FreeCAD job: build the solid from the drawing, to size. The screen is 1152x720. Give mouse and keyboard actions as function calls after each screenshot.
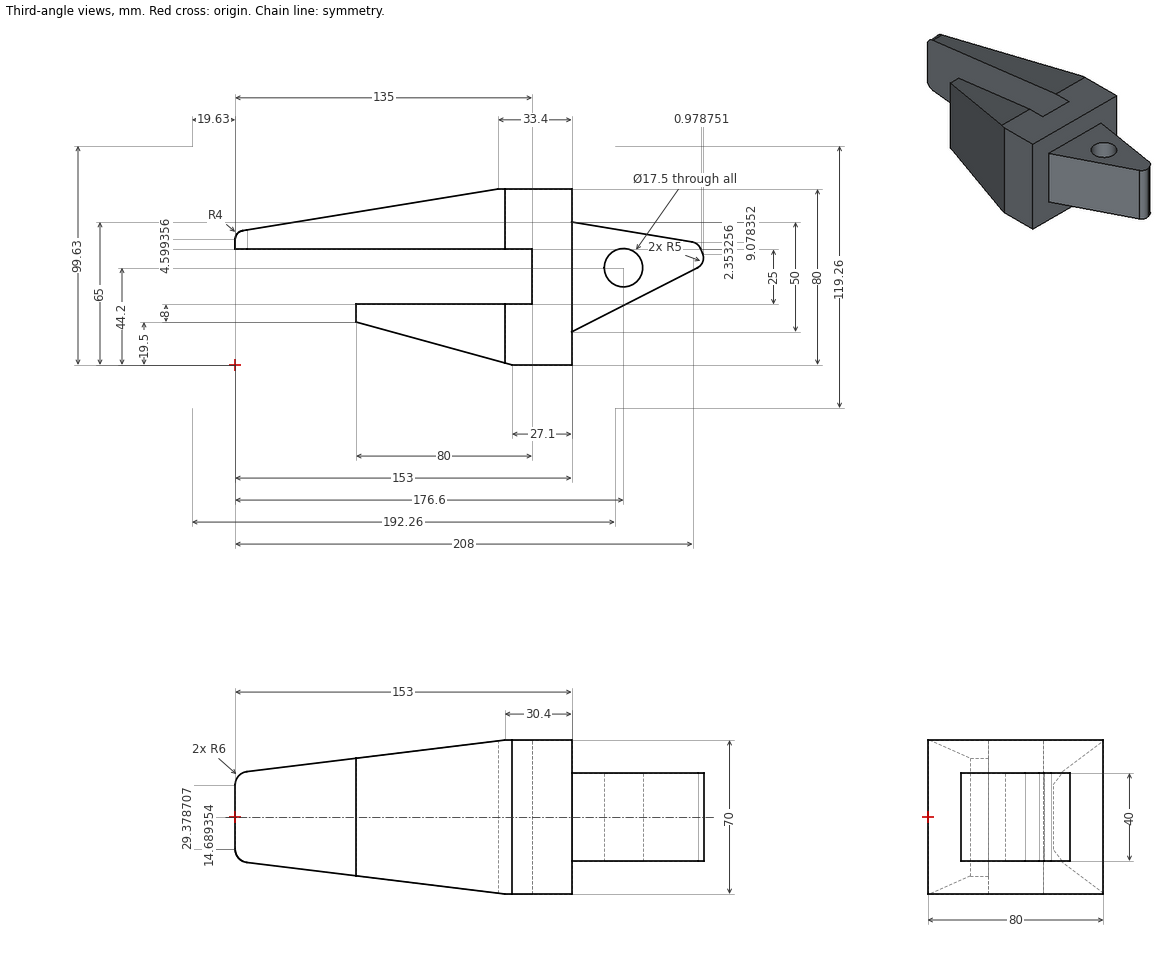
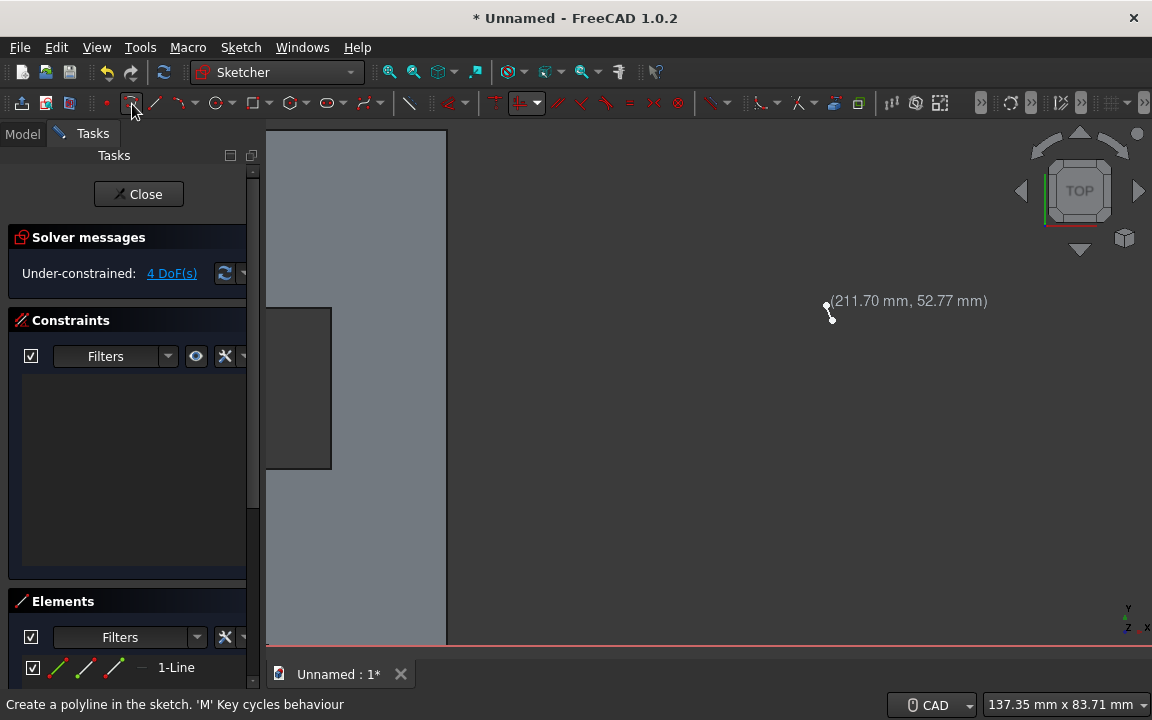
click(801, 286)
click(447, 227)
click(447, 550)
click(817, 361)
right_click(817, 361)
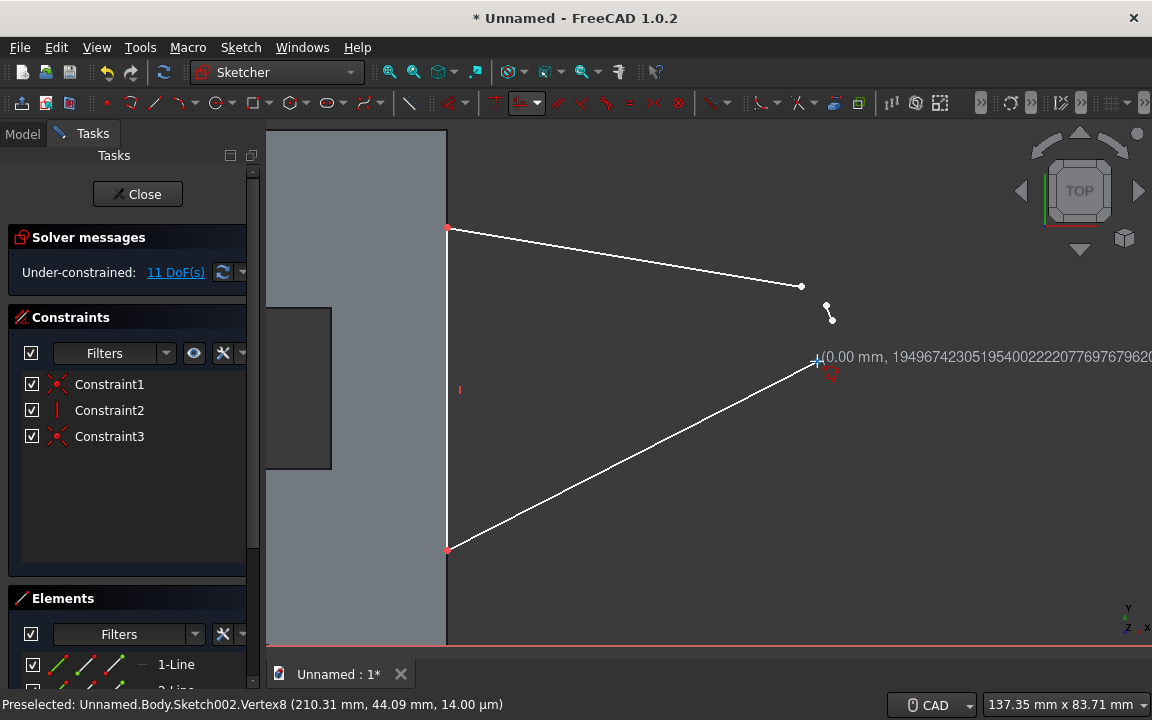
click(180, 104)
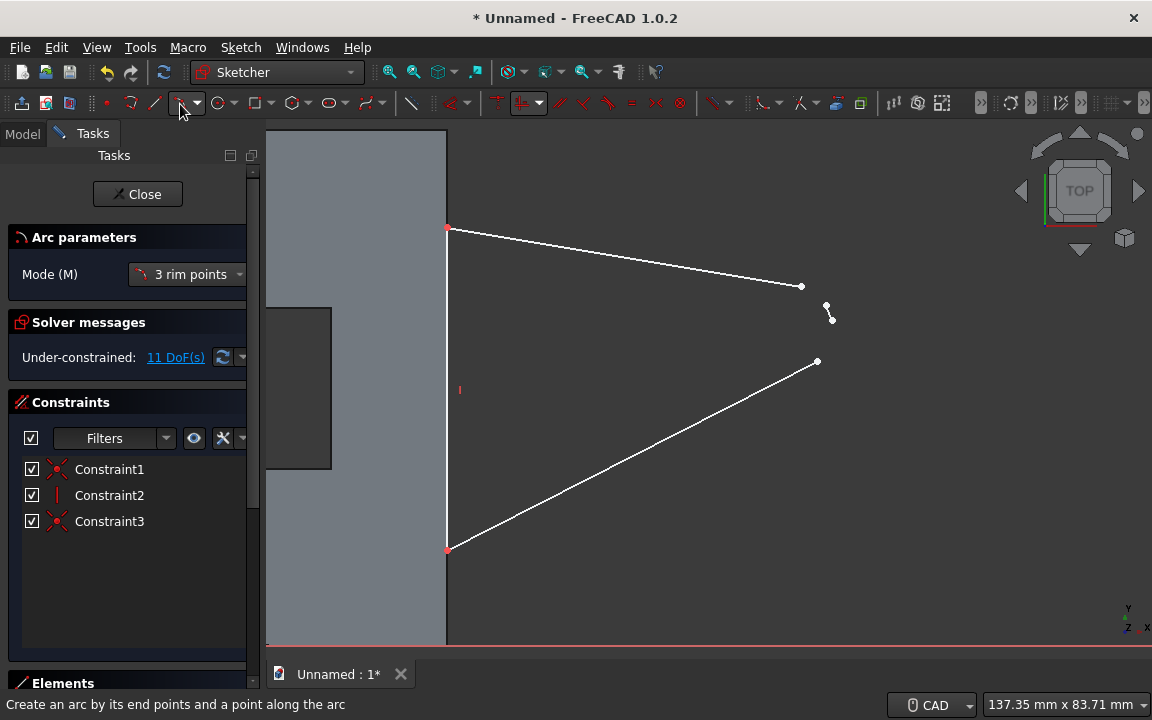
scroll(826, 305, up, 4)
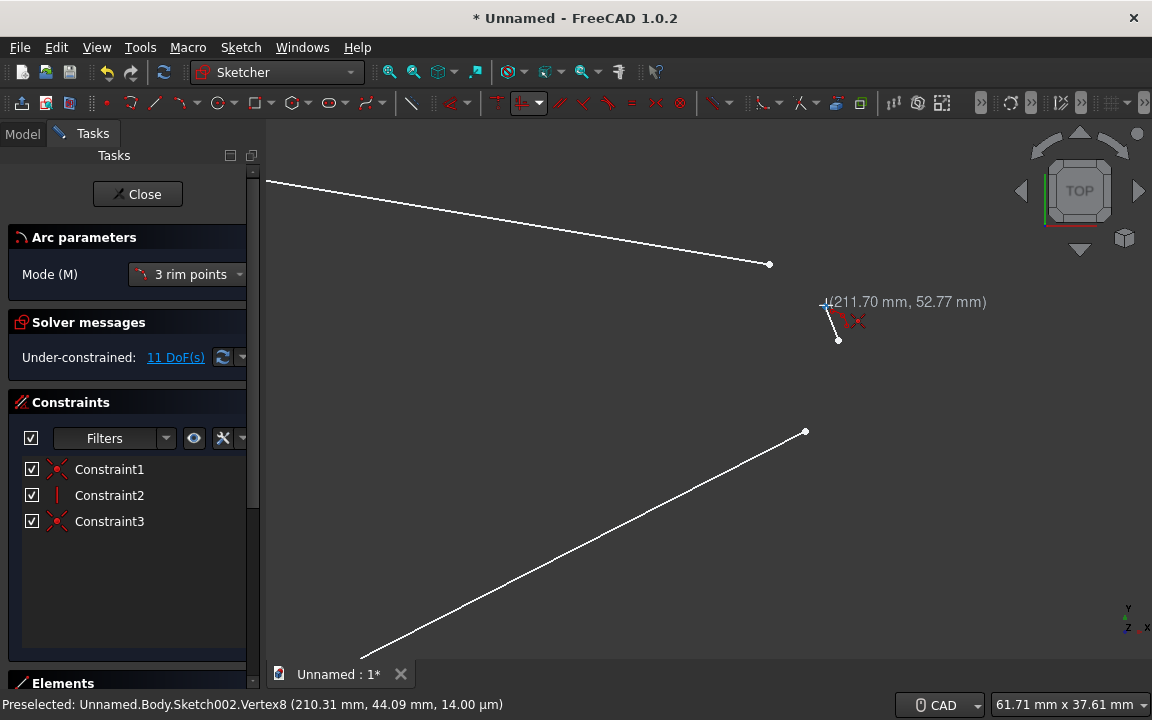
click(825, 307)
click(770, 265)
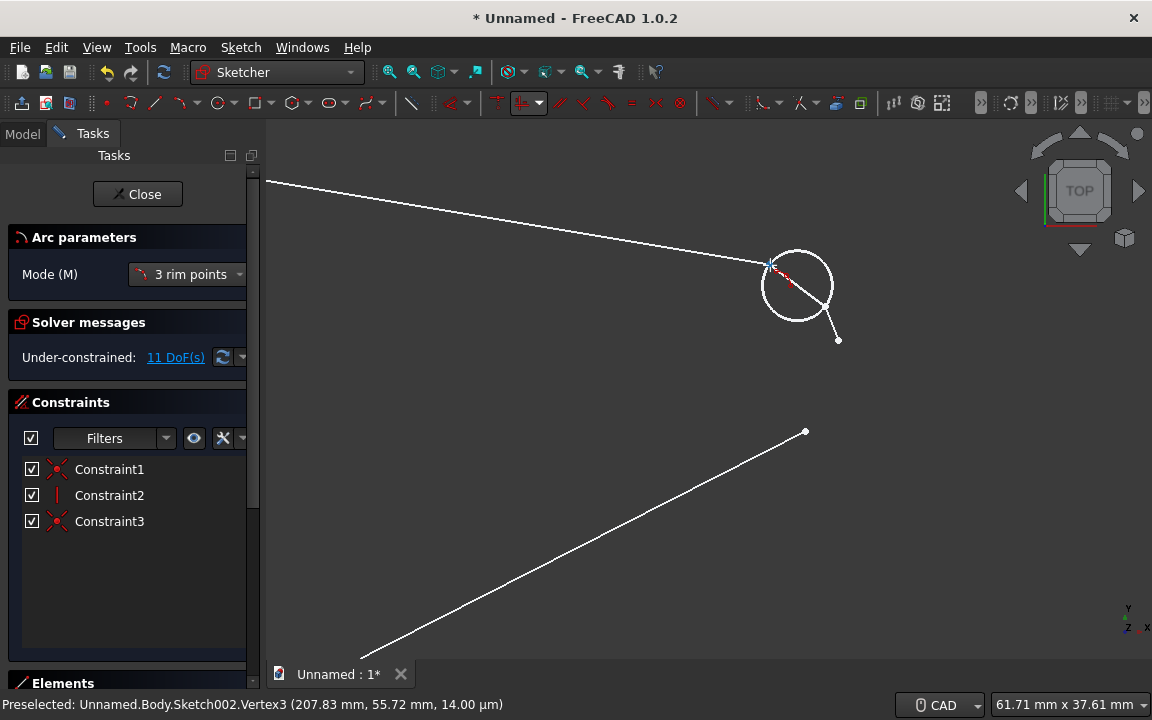
scroll(803, 276, up, 3)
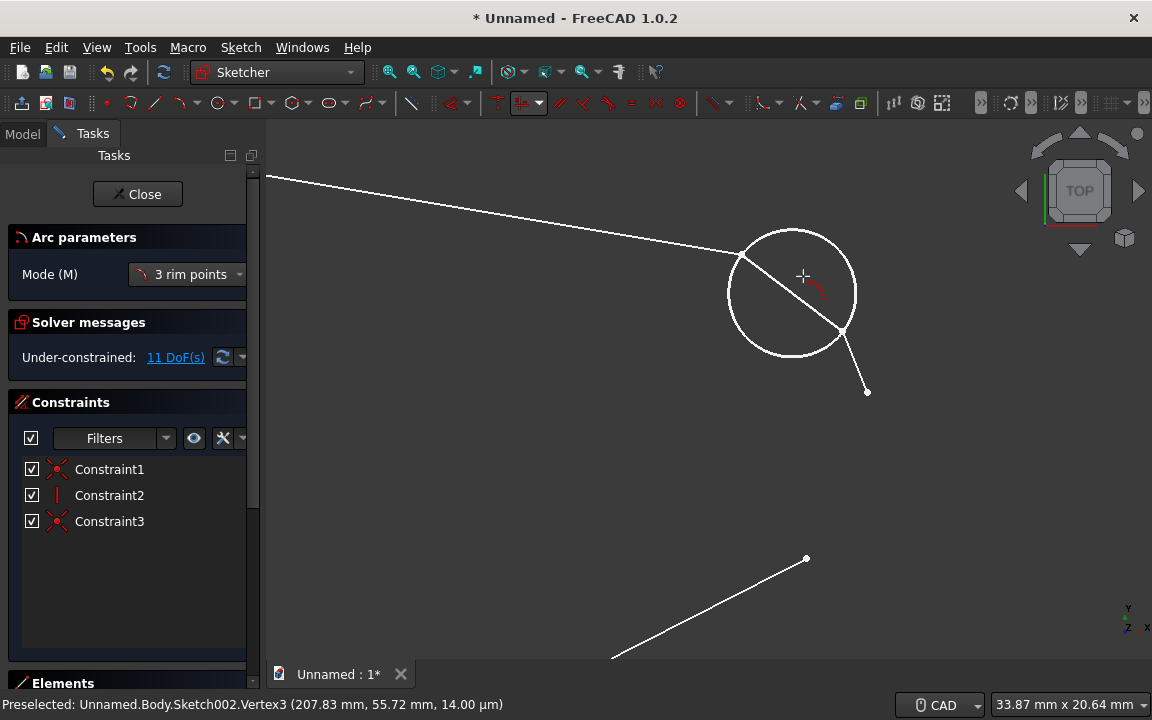
click(802, 276)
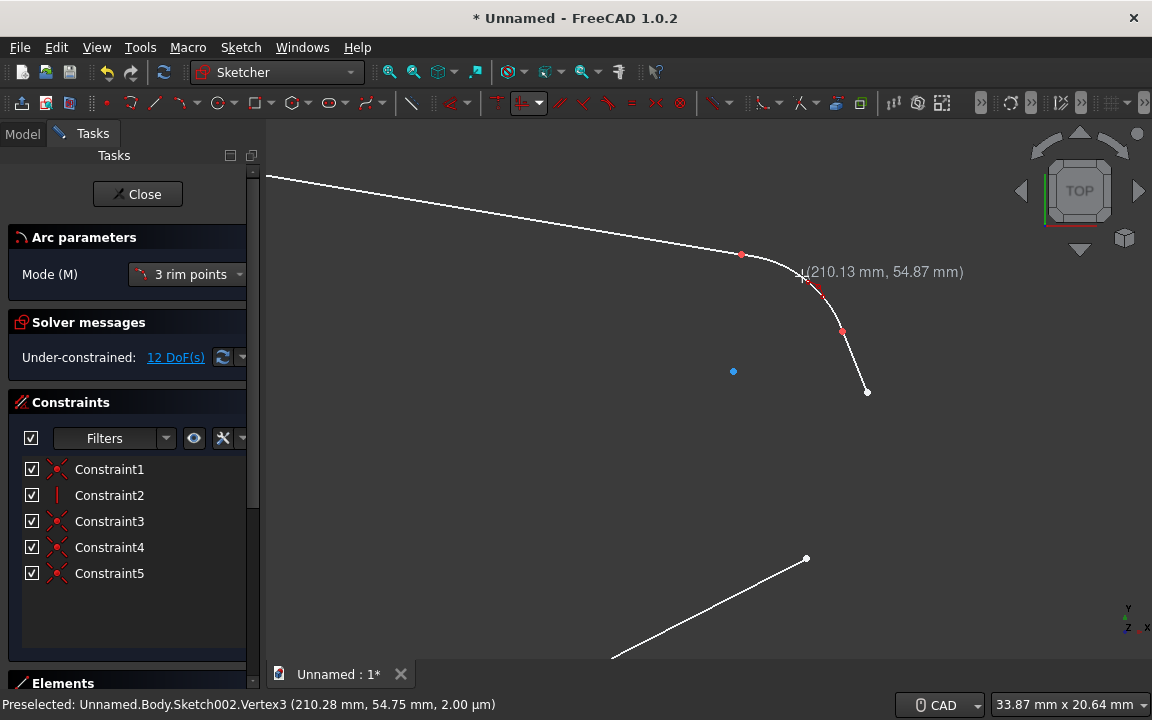
scroll(821, 298, down, 7)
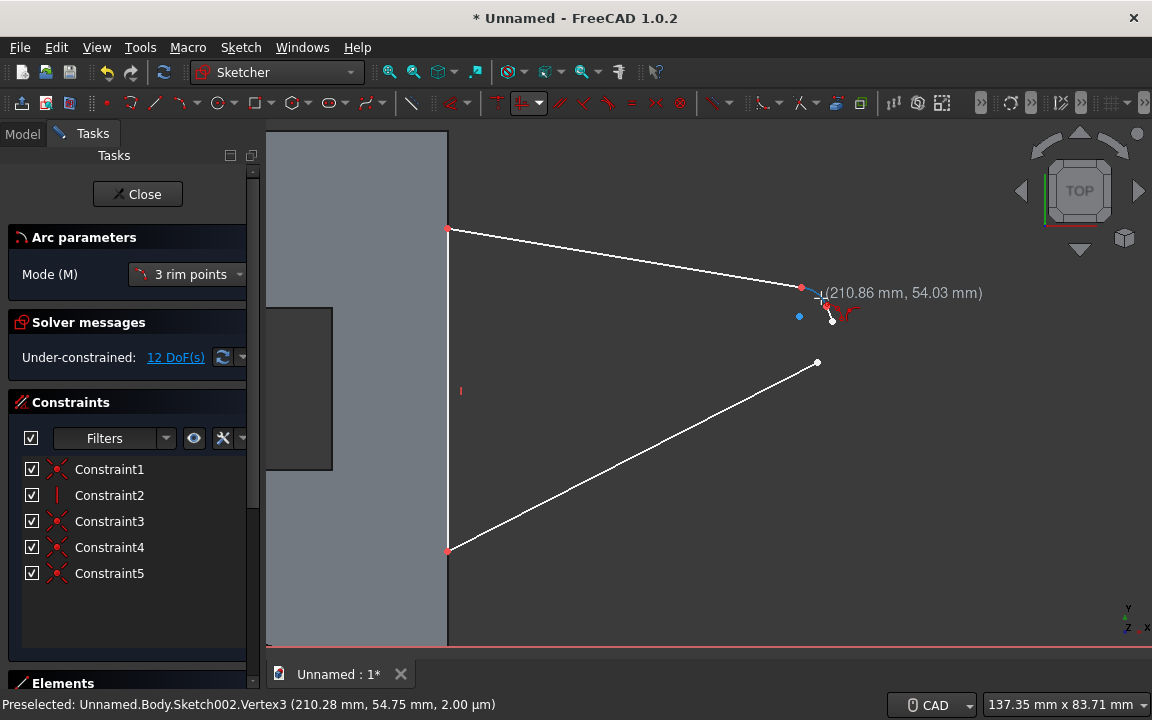
click(818, 363)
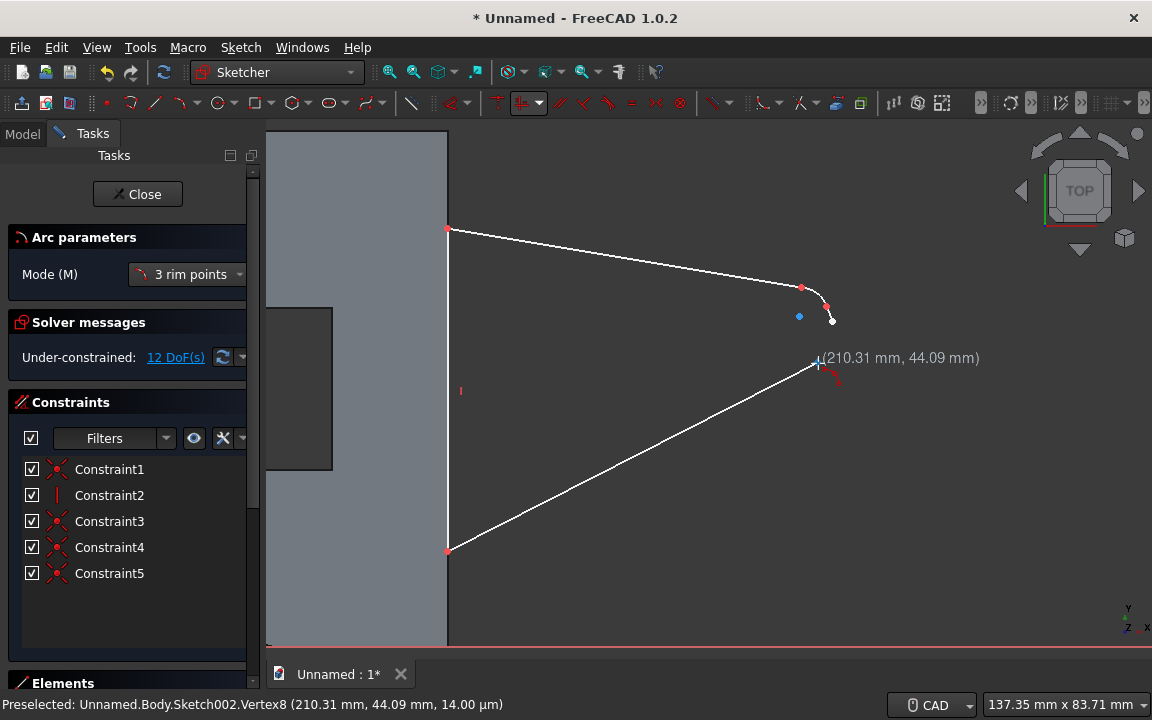
scroll(833, 321, up, 4)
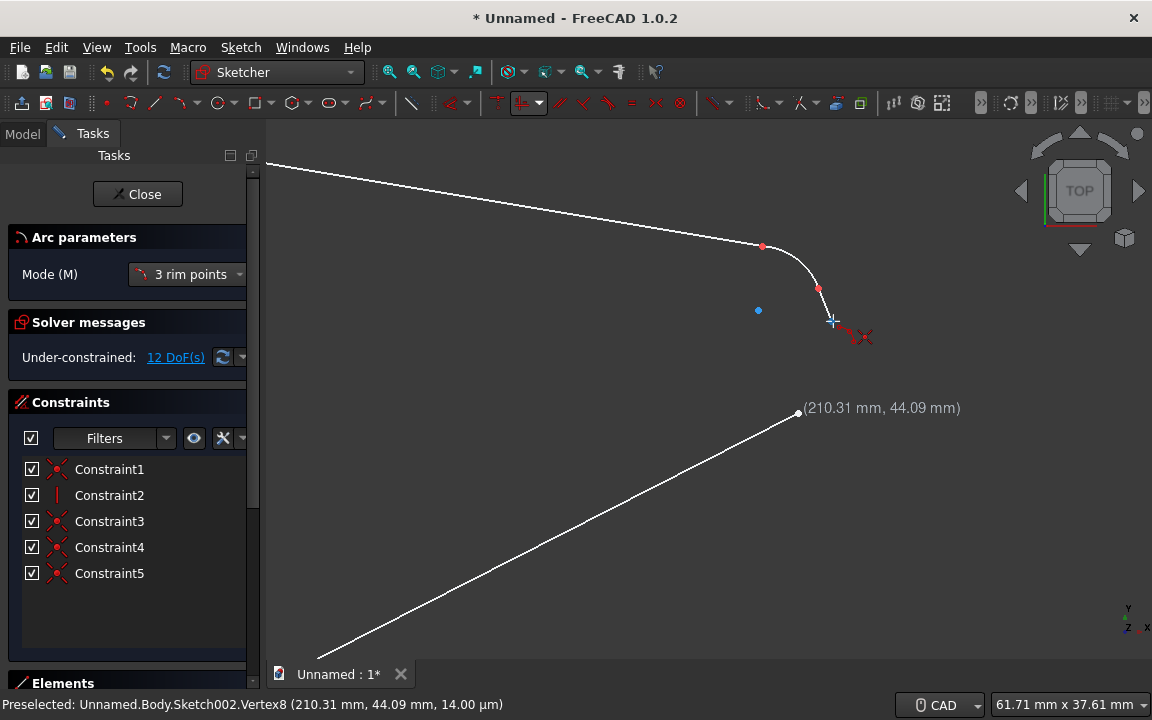
click(832, 322)
click(833, 373)
key(Escape)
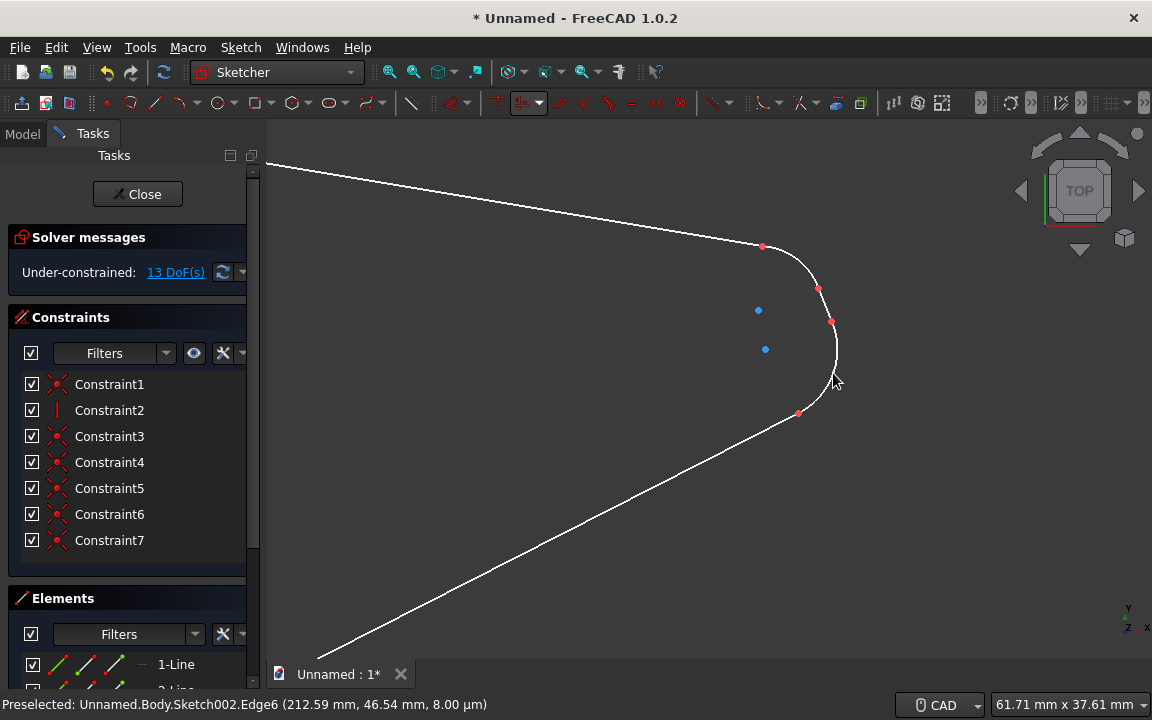
scroll(828, 312, up, 2)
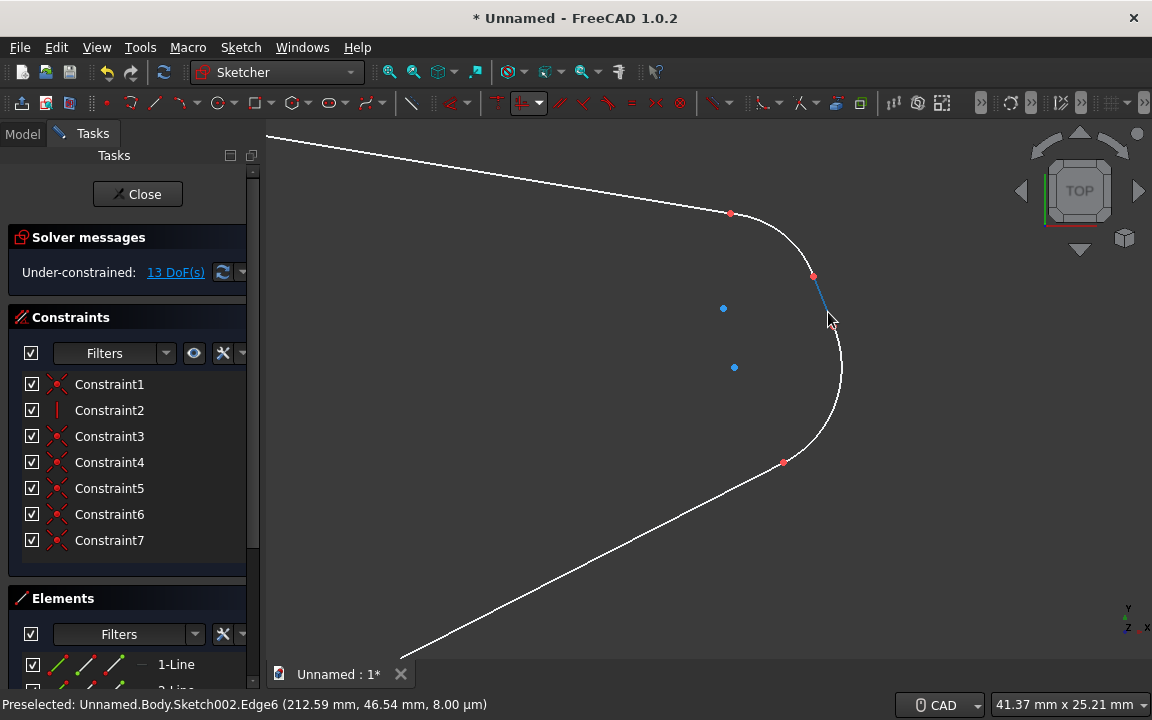
click(828, 312)